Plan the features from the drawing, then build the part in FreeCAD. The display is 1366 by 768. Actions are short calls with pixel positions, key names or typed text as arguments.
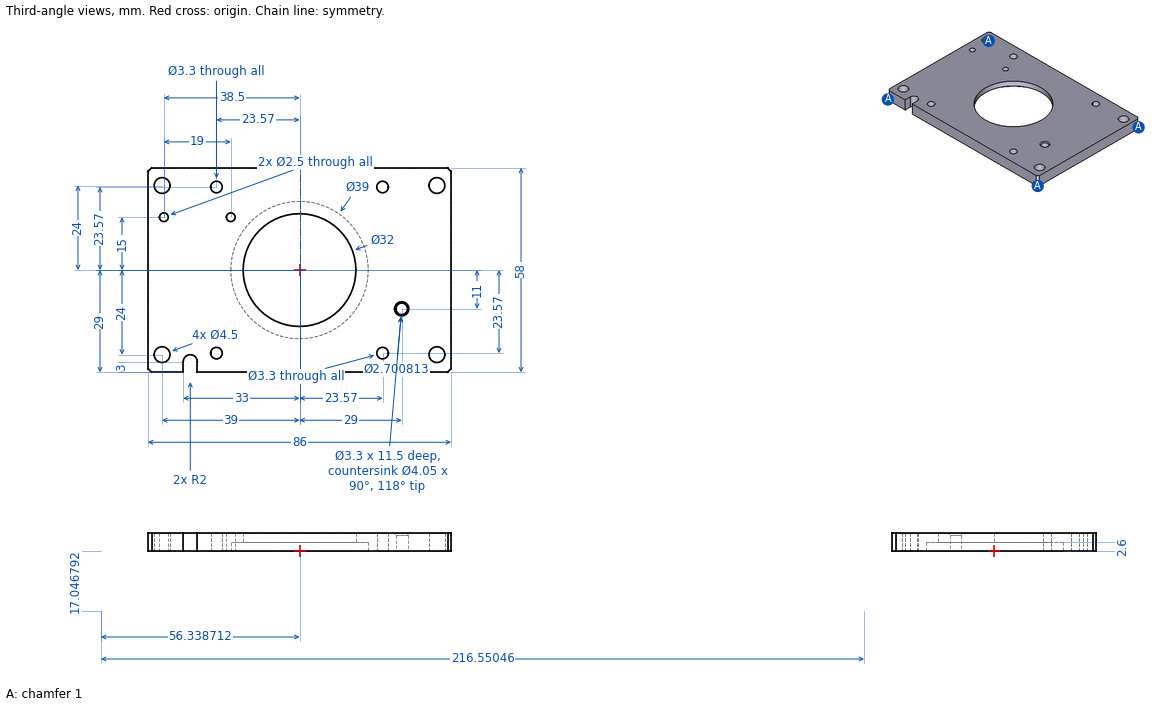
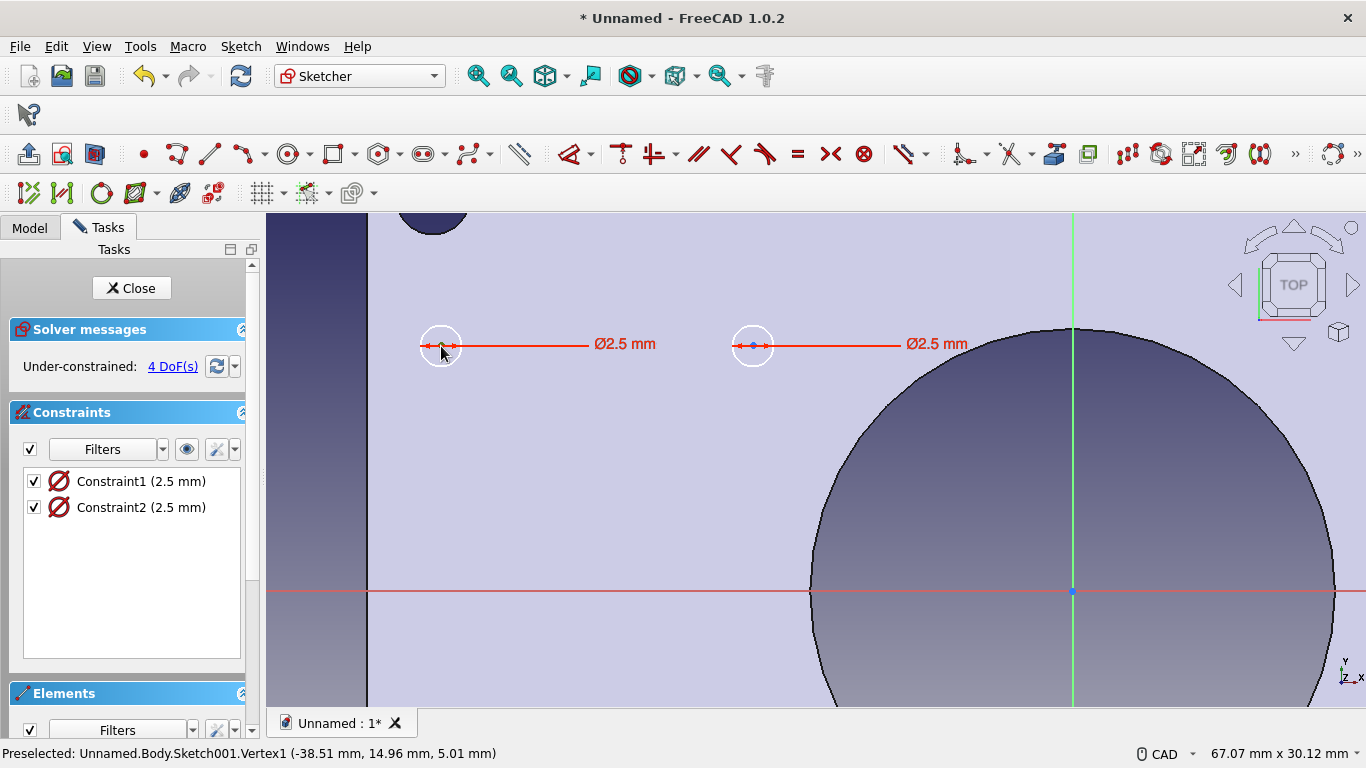
click(753, 346)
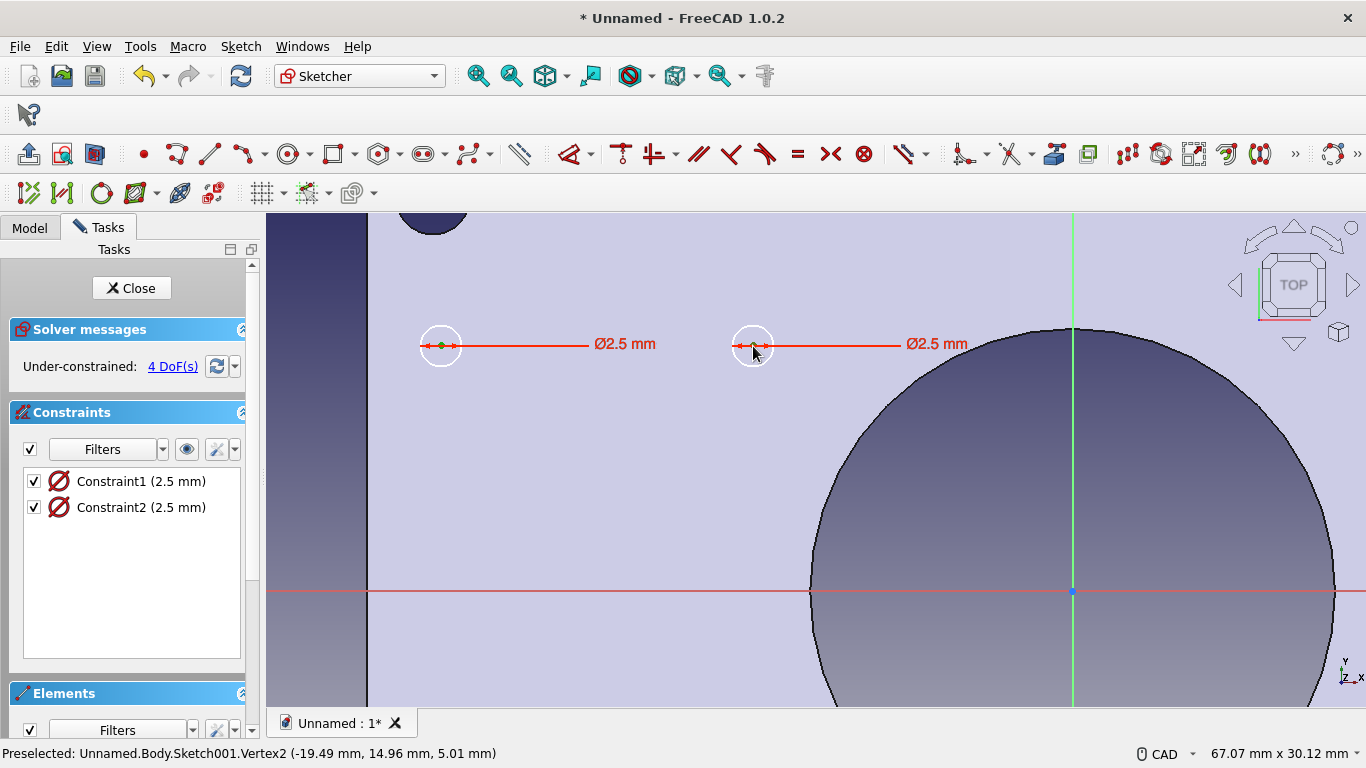
key(h)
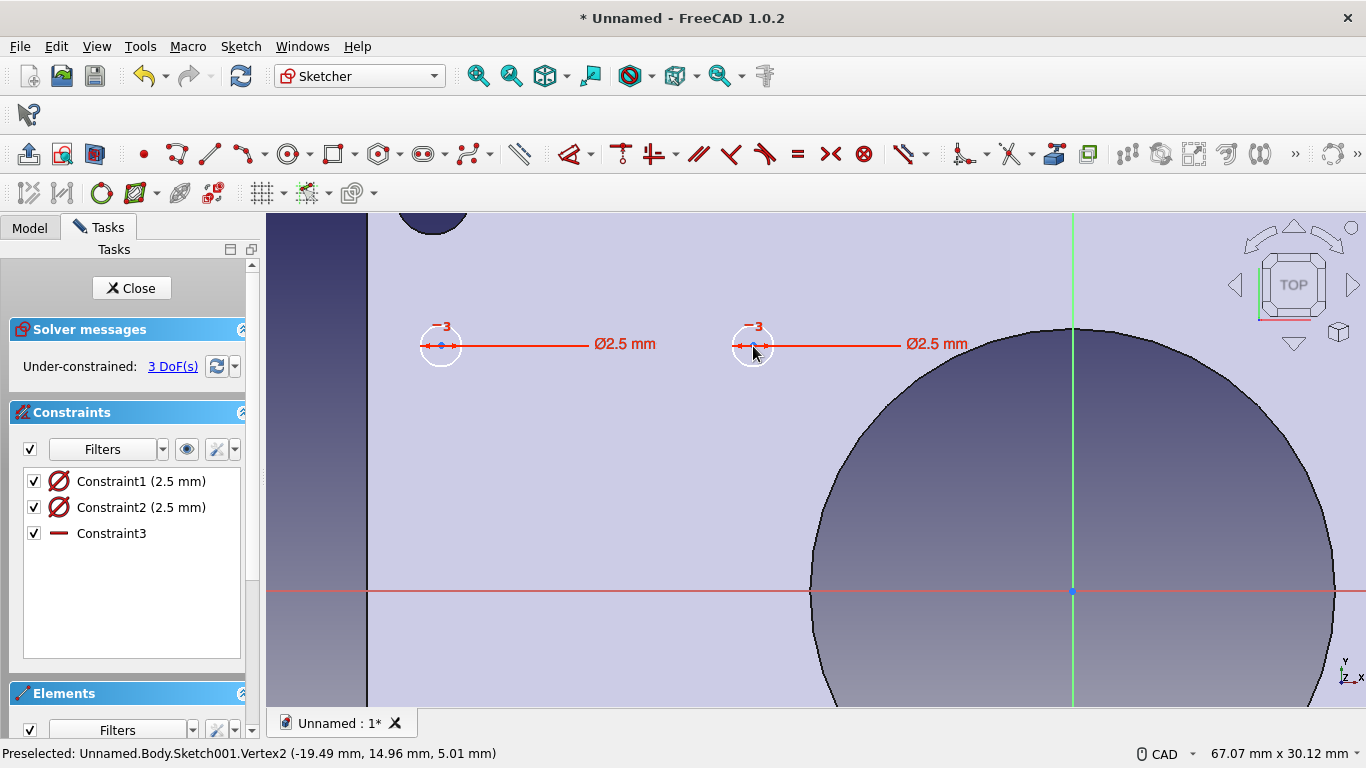
key(d)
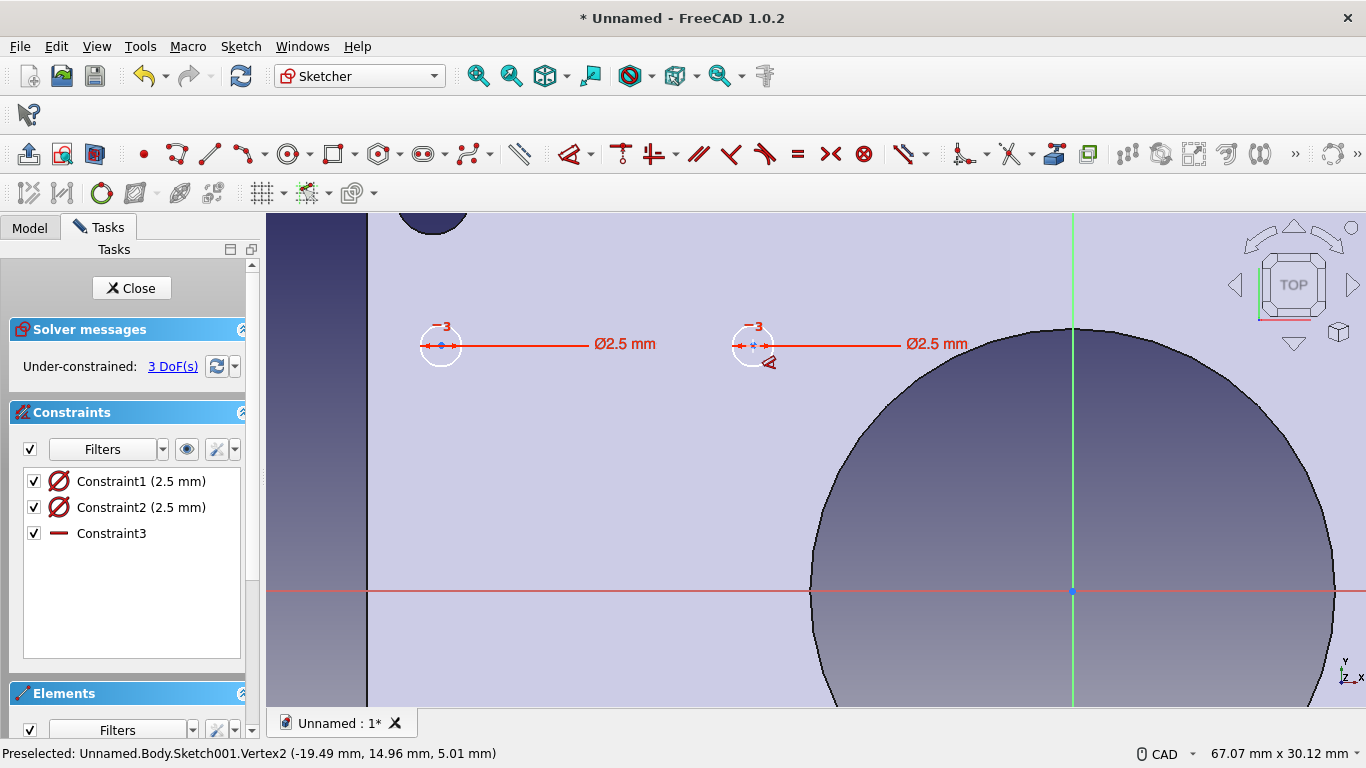
click(441, 346)
click(1107, 469)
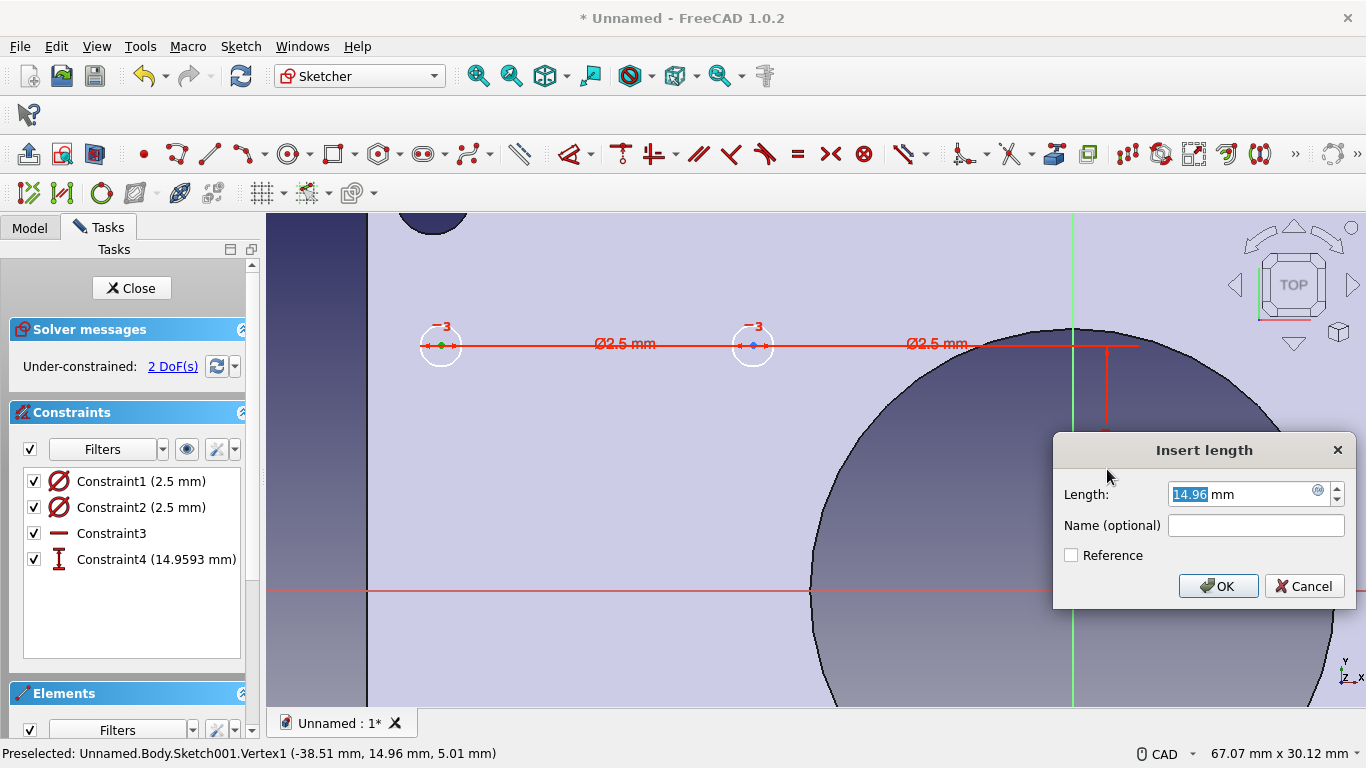
text(15)
key(Return)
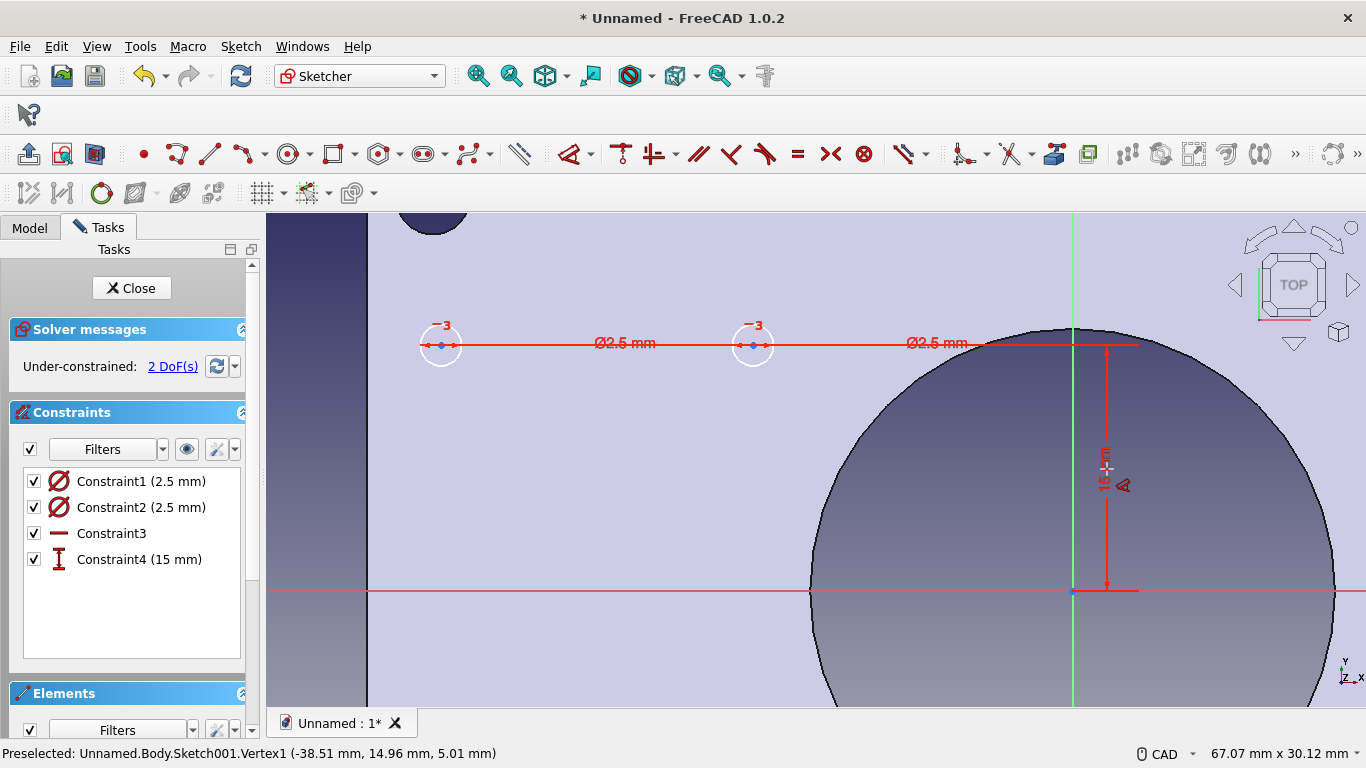
click(441, 345)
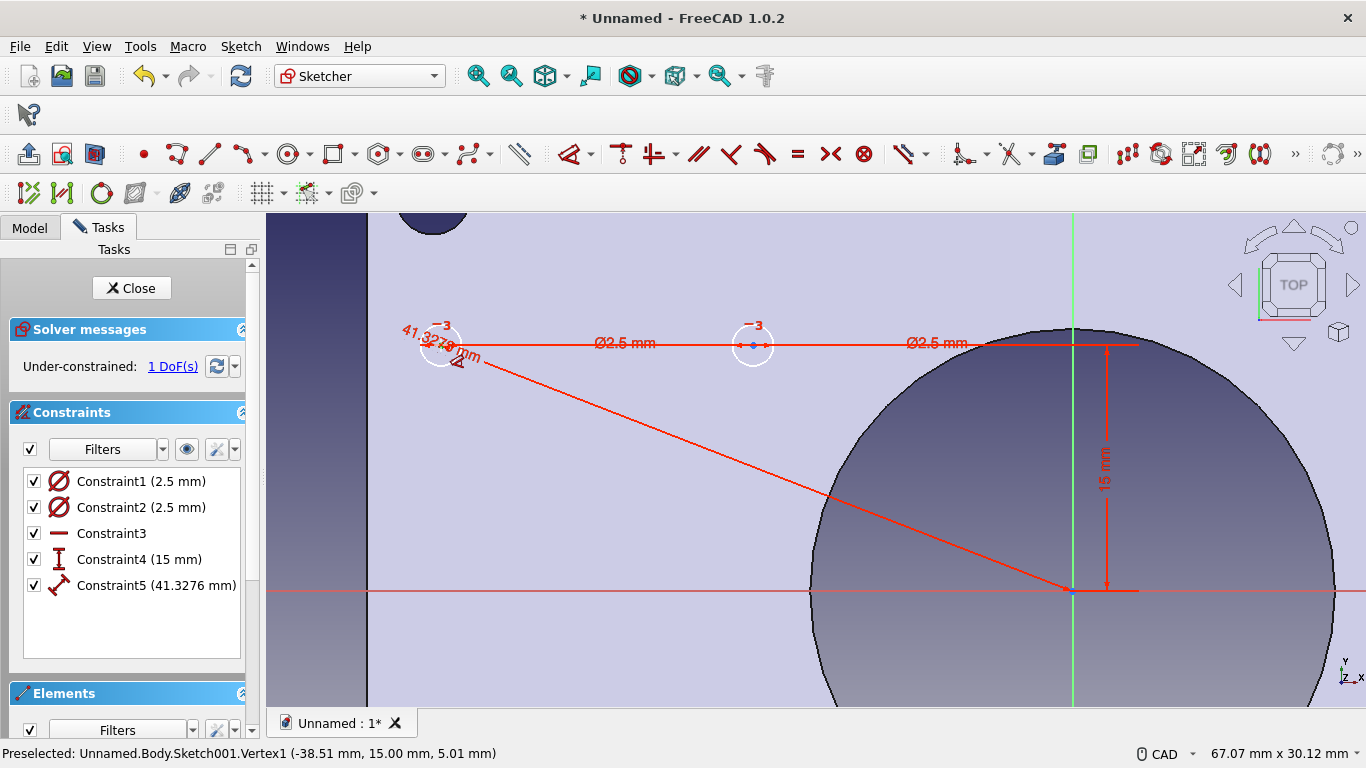
click(753, 345)
click(597, 311)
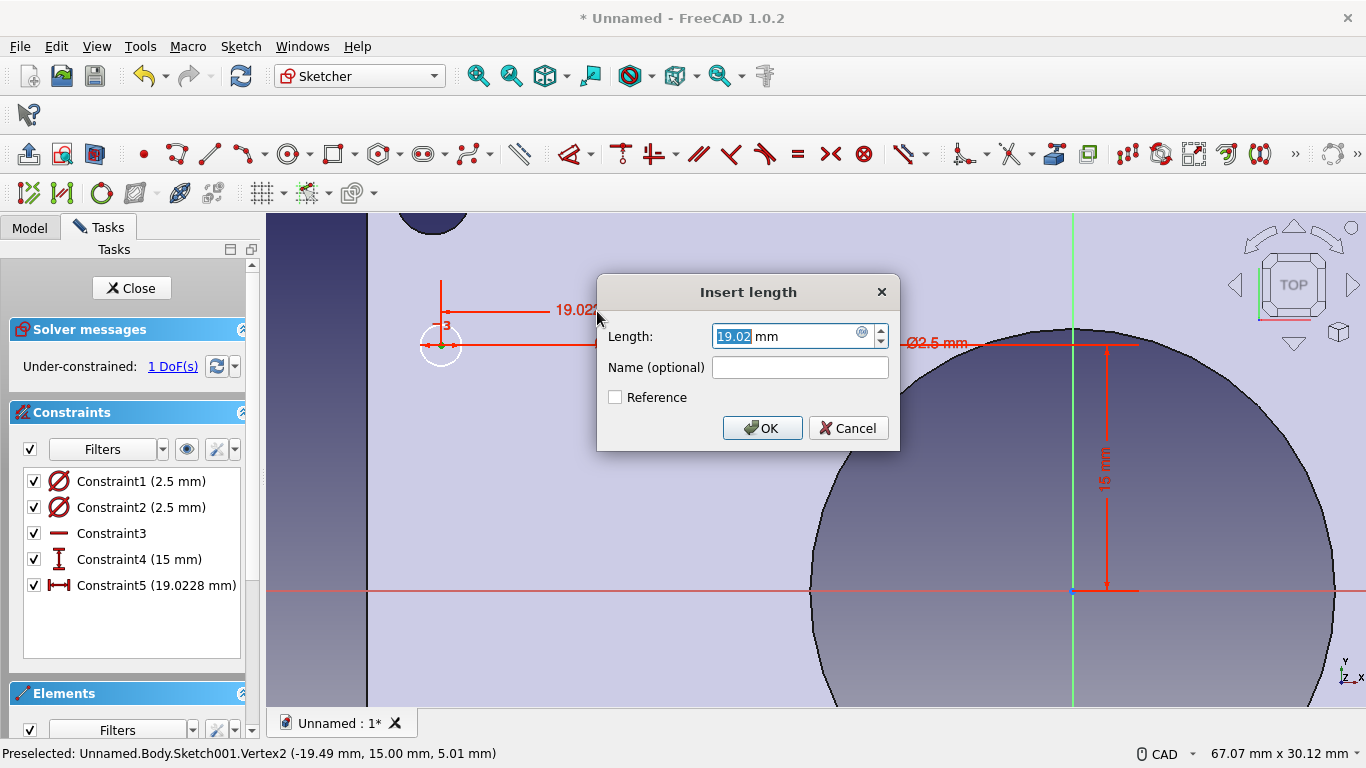
text(19)
key(Return)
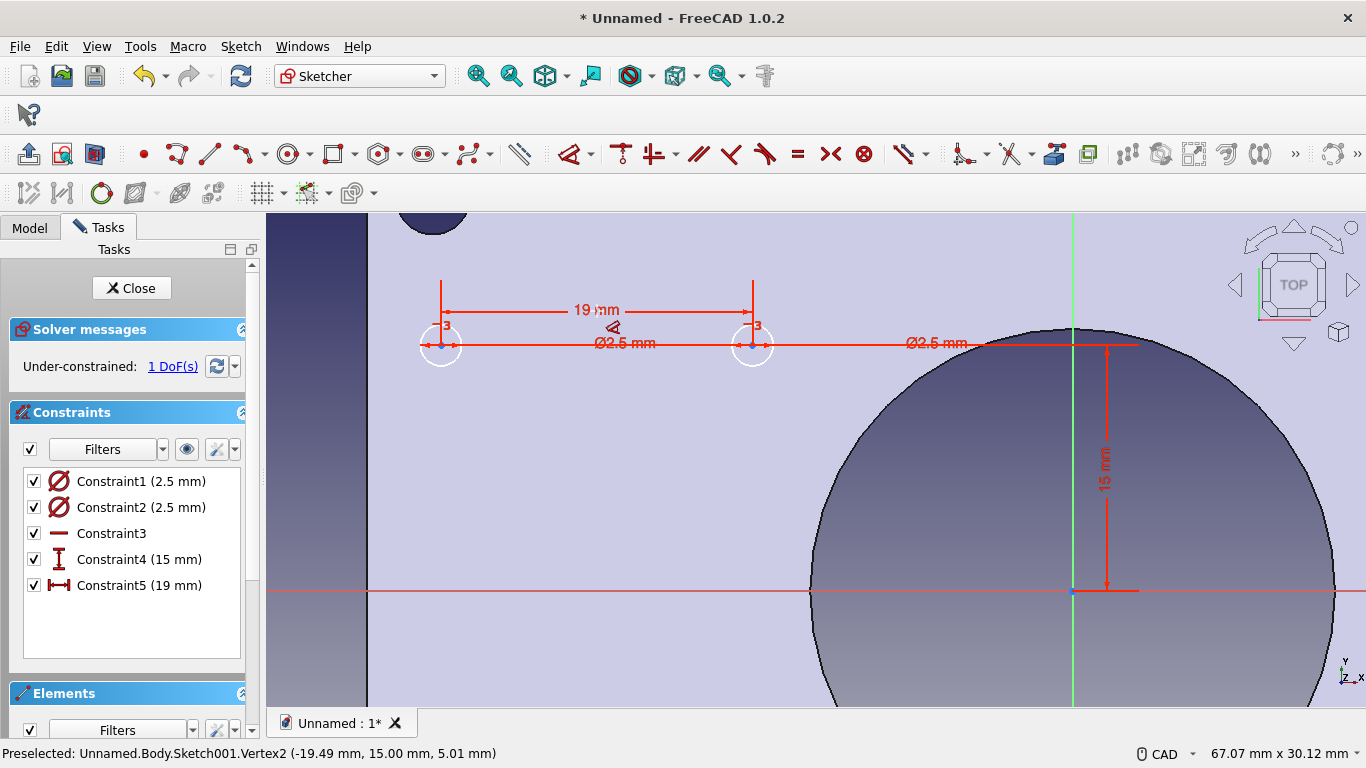
click(441, 345)
click(757, 625)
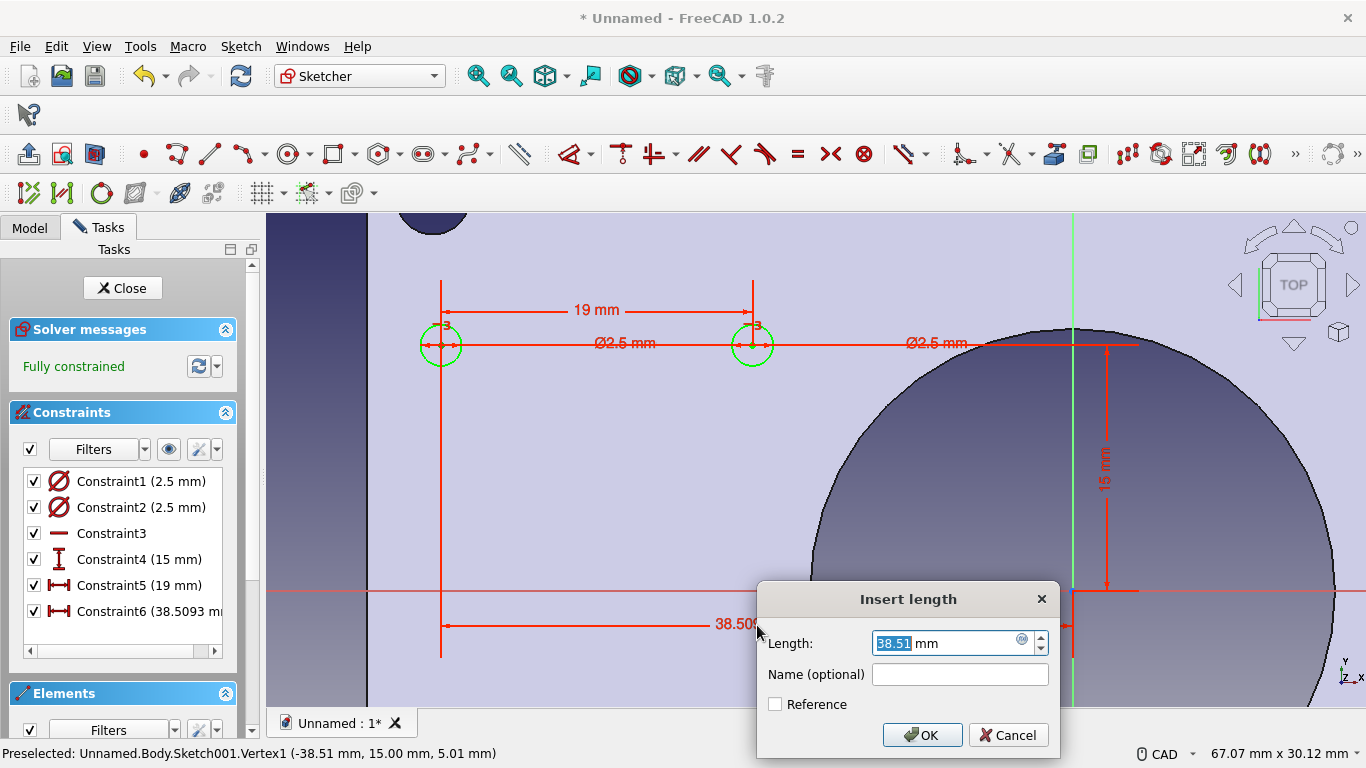
text(38.5)
key(Return)
key(Escape)